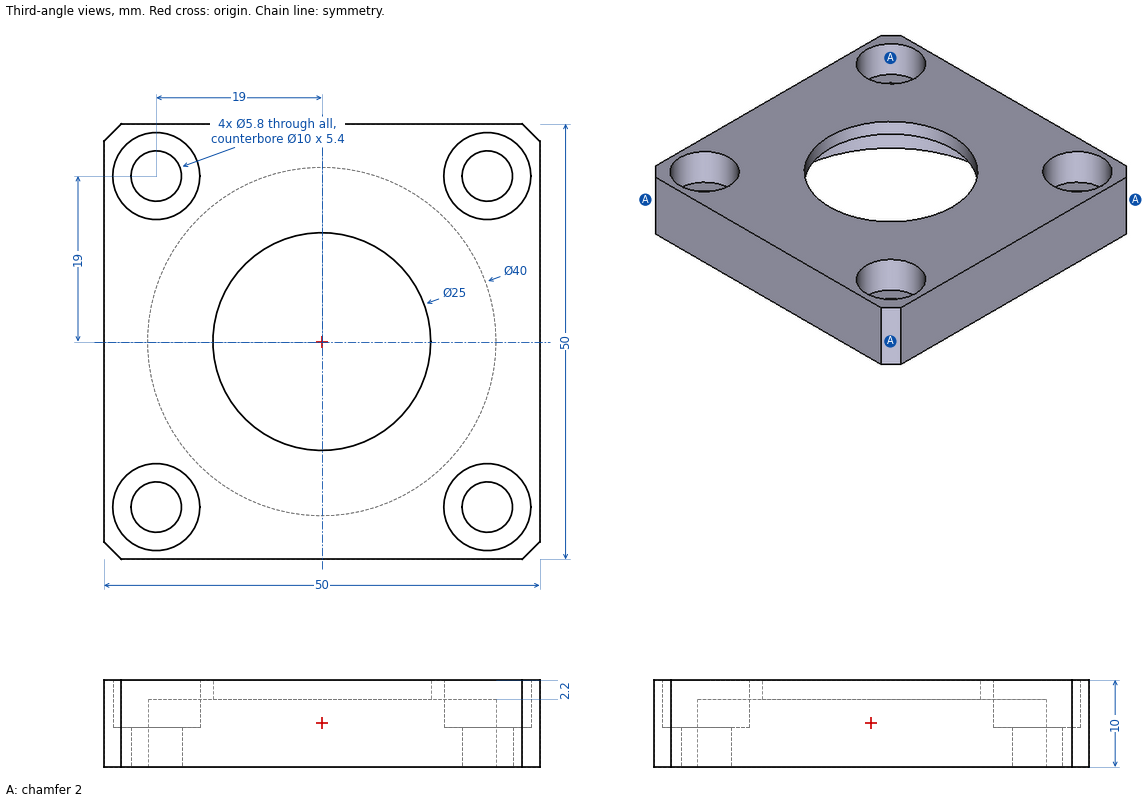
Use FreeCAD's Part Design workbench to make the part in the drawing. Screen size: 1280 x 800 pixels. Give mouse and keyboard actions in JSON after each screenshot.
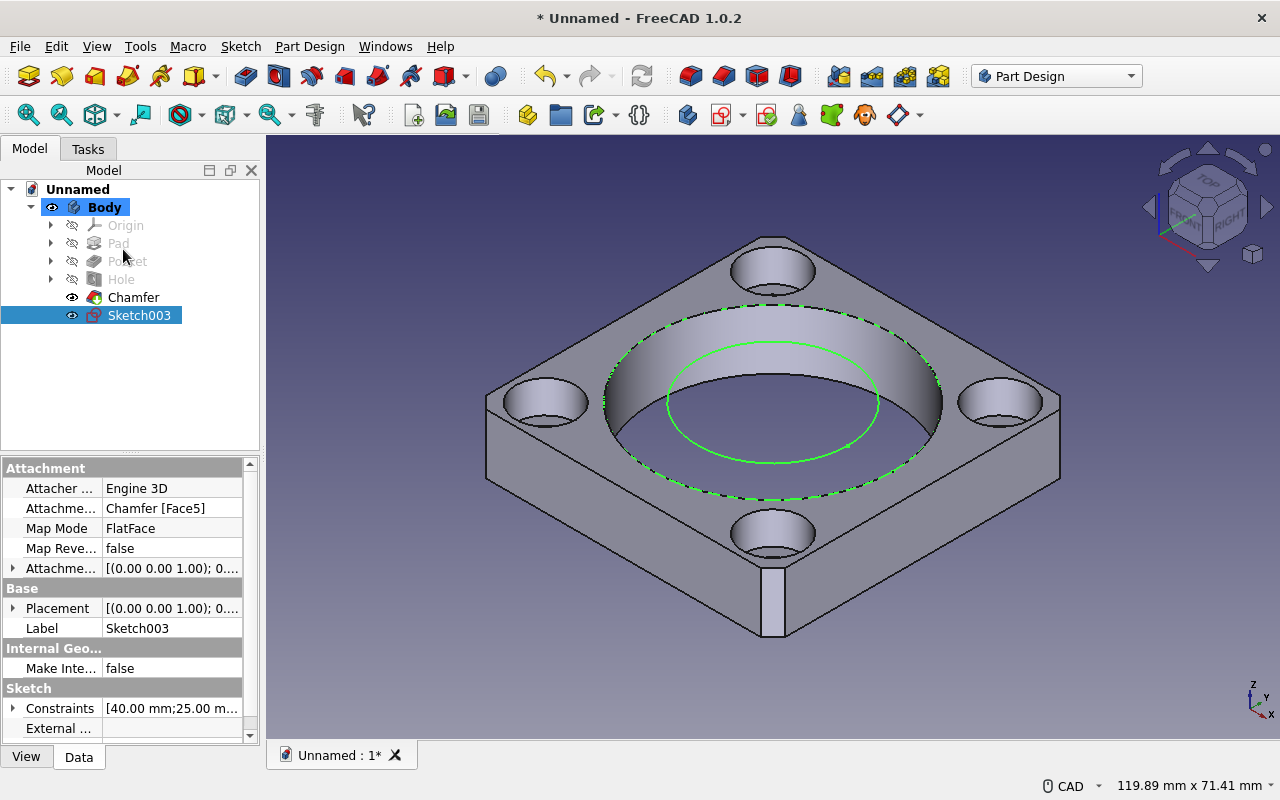
{"action": "left_click", "coordinate": [29, 76]}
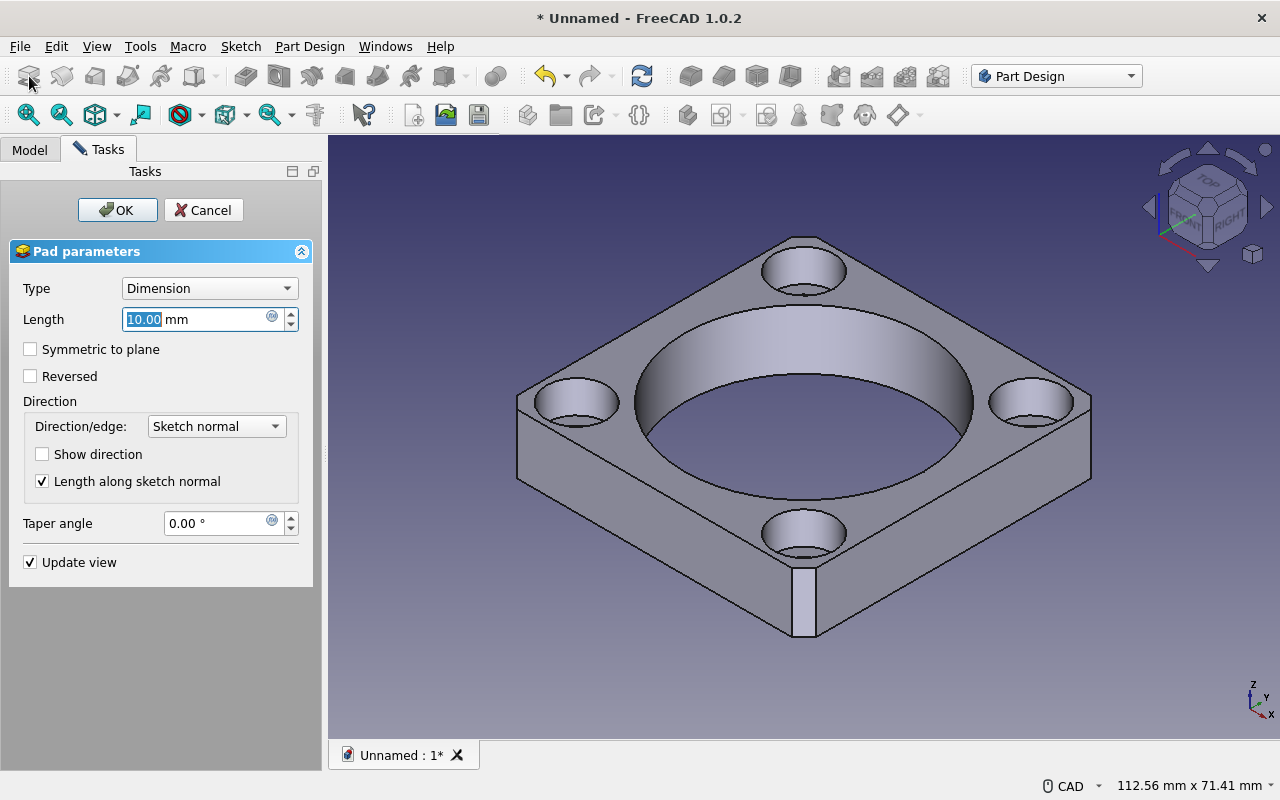
{"action": "type", "text": "2.2"}
{"action": "key", "text": "Tab"}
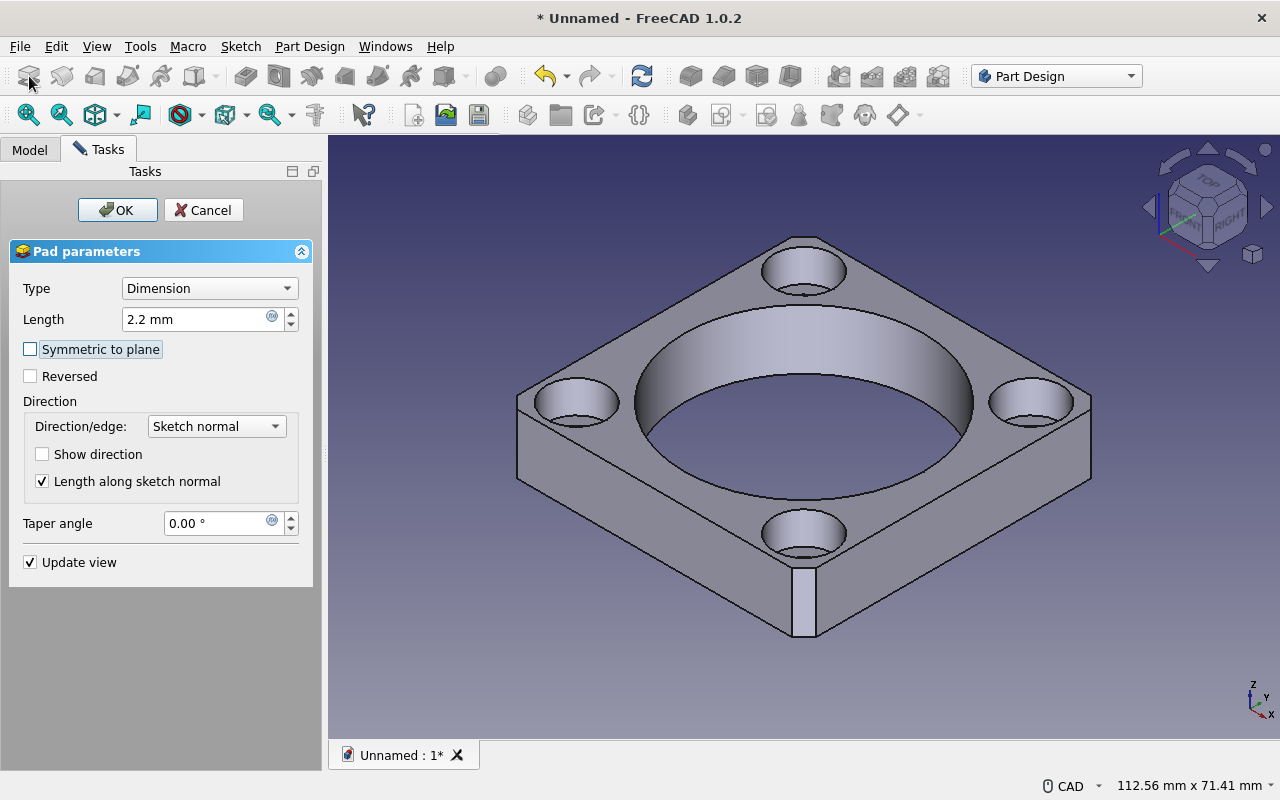
{"action": "left_click", "coordinate": [31, 376]}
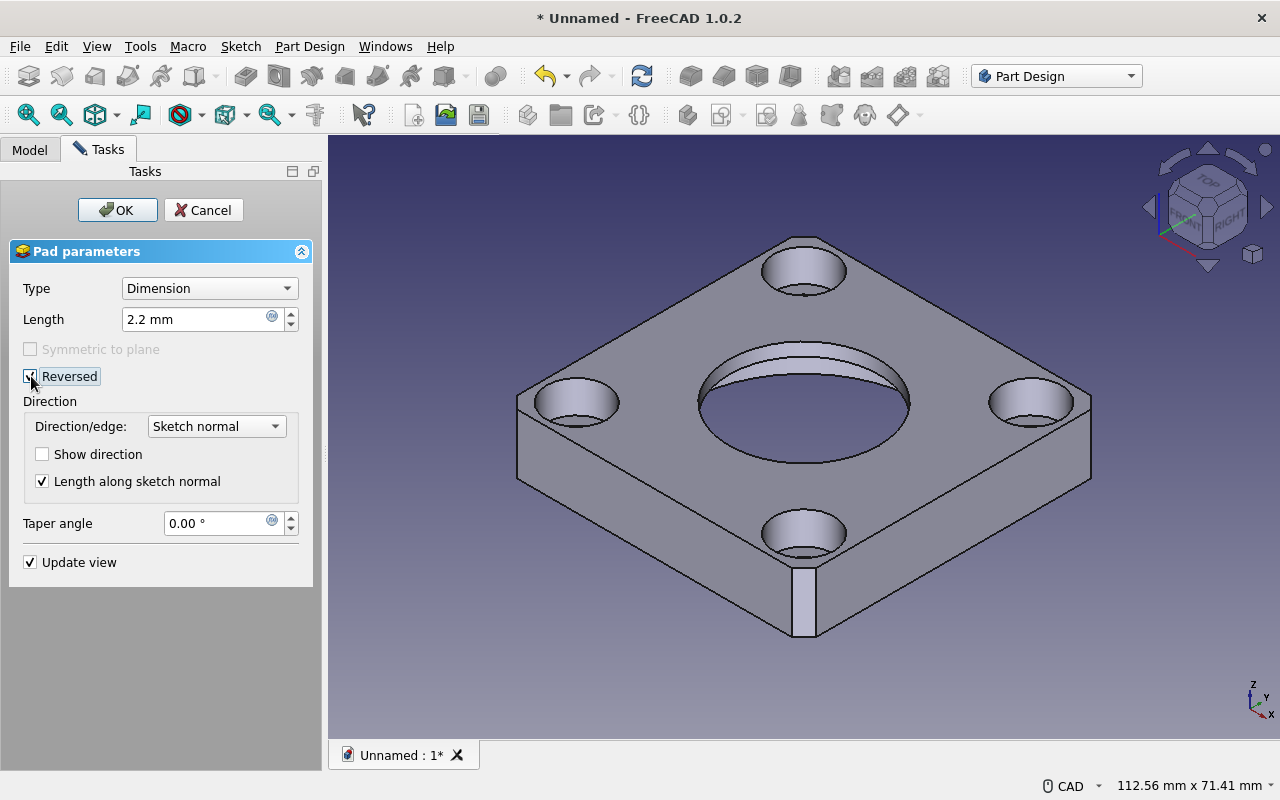
{"action": "left_click", "coordinate": [118, 210]}